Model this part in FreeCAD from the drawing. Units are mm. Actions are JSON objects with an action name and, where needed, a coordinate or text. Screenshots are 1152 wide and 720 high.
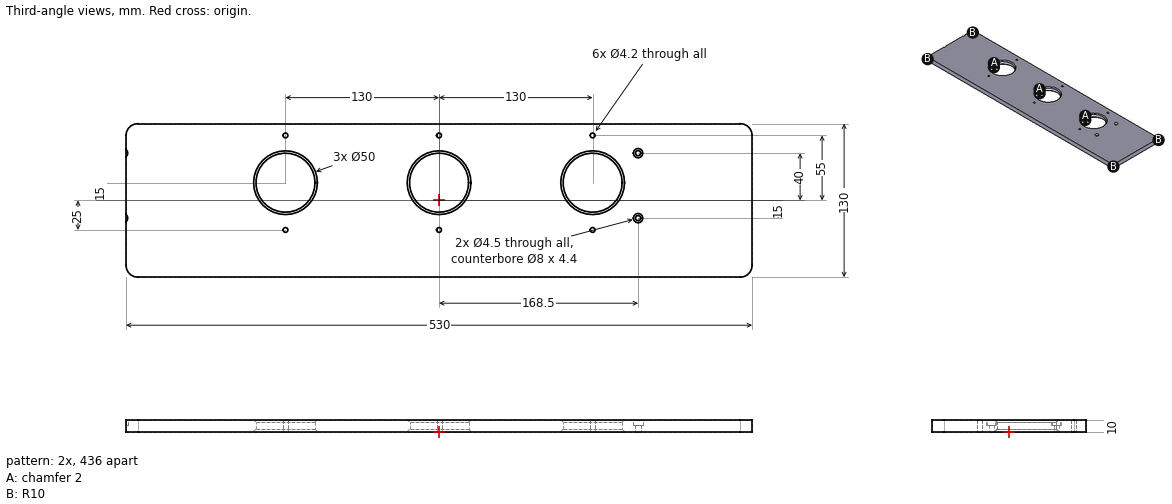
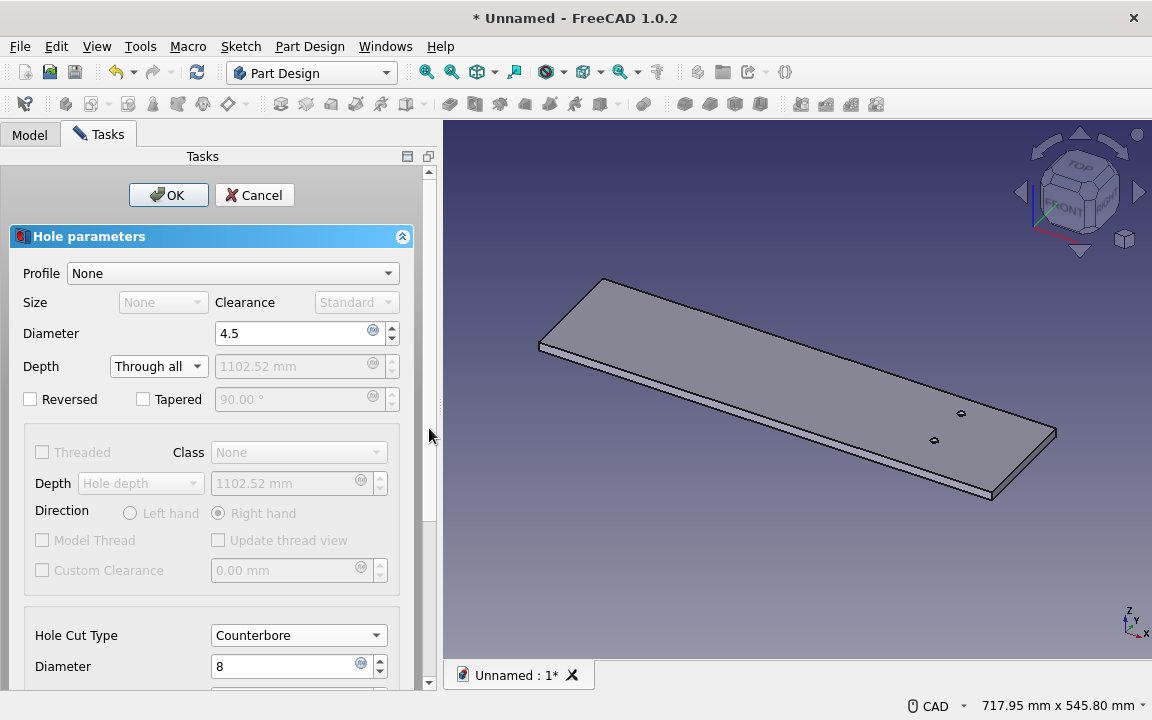
{"action": "left_click", "coordinate": [169, 195]}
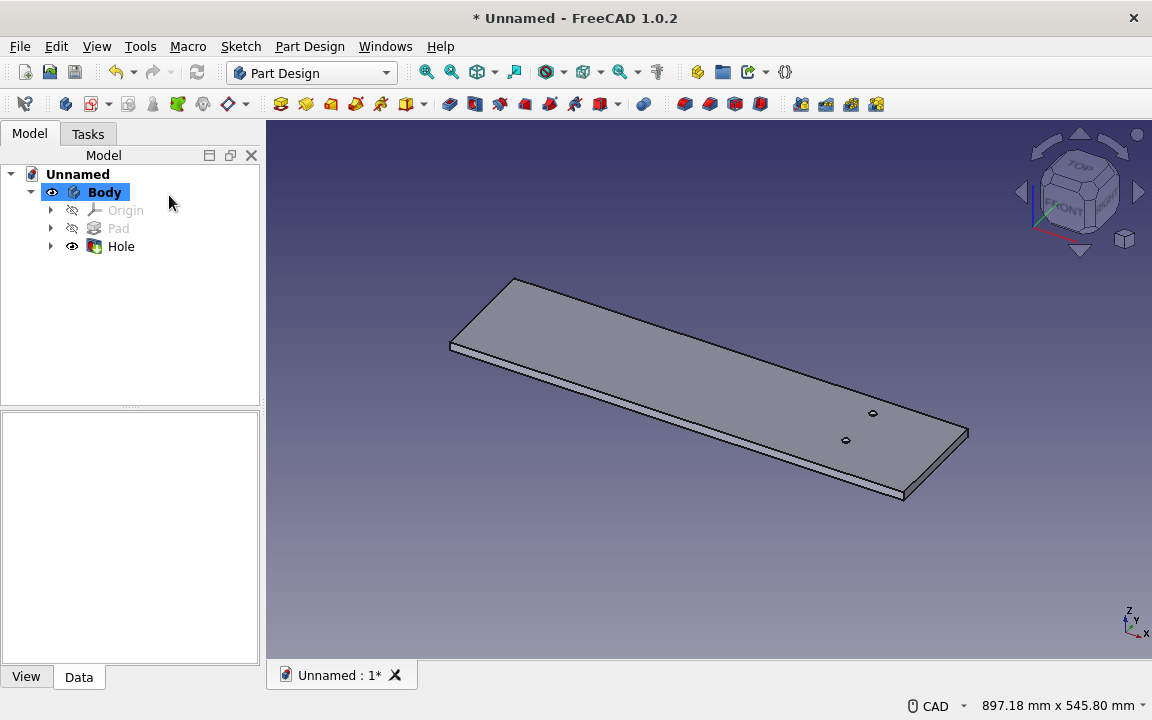
{"action": "left_click", "coordinate": [117, 246]}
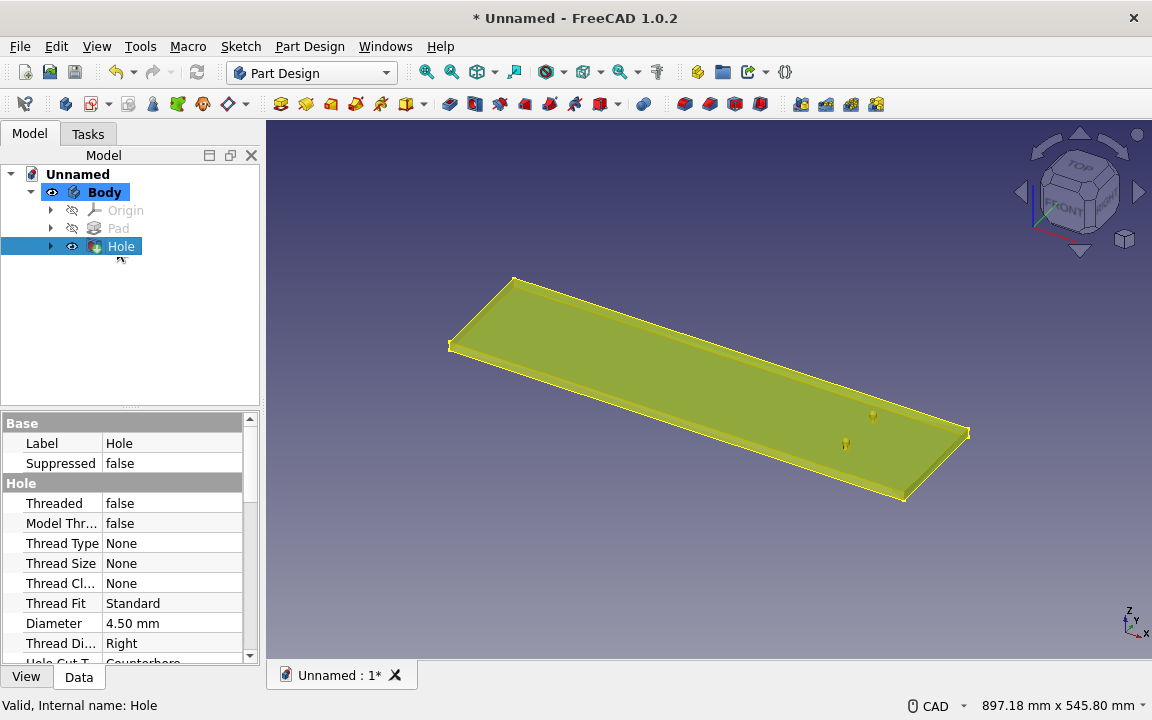
{"action": "left_click", "coordinate": [826, 104]}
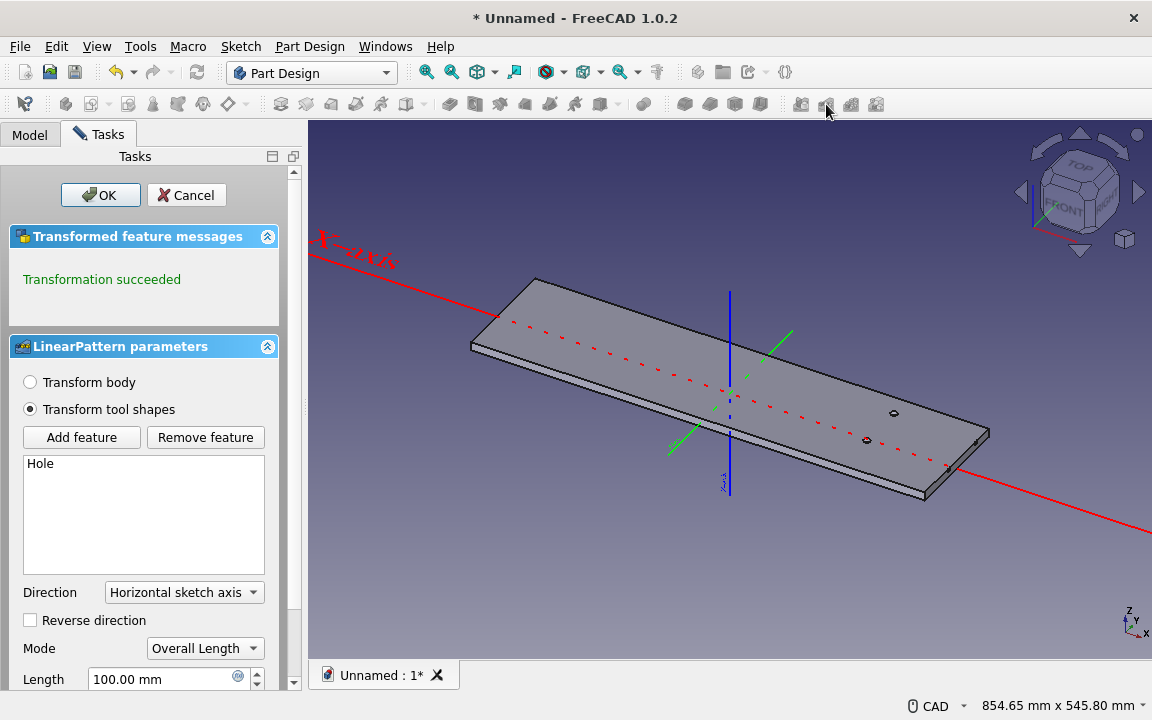
{"action": "left_click", "coordinate": [185, 592]}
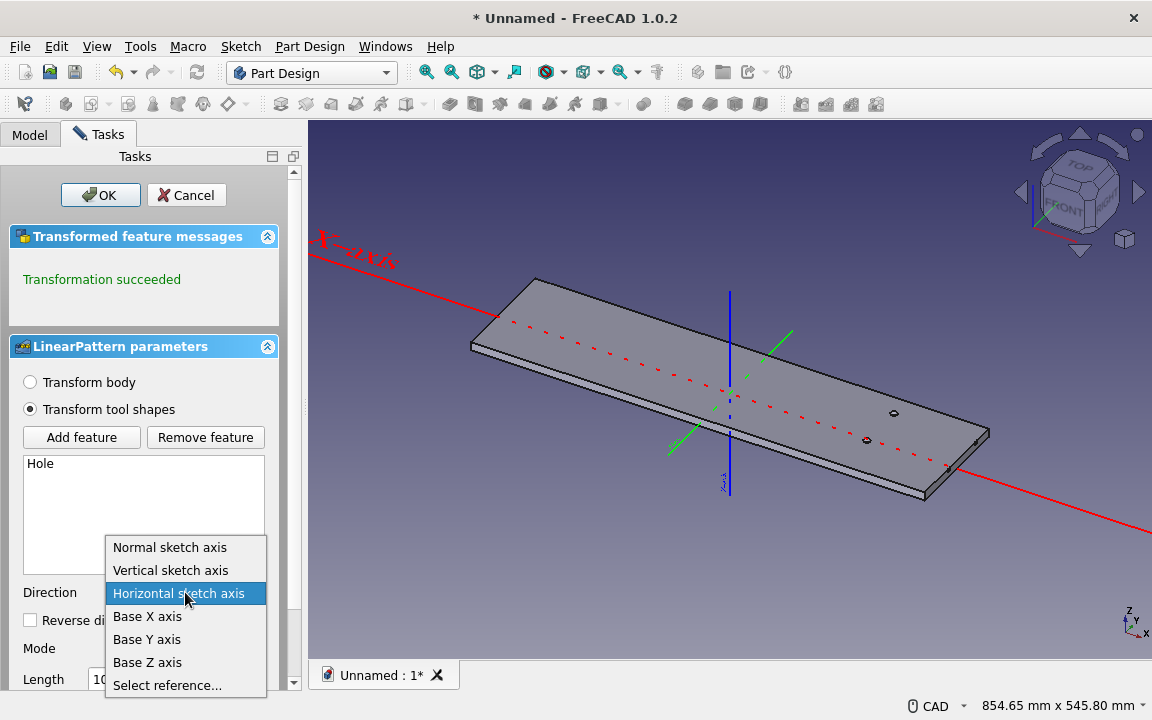
{"action": "left_click", "coordinate": [184, 616]}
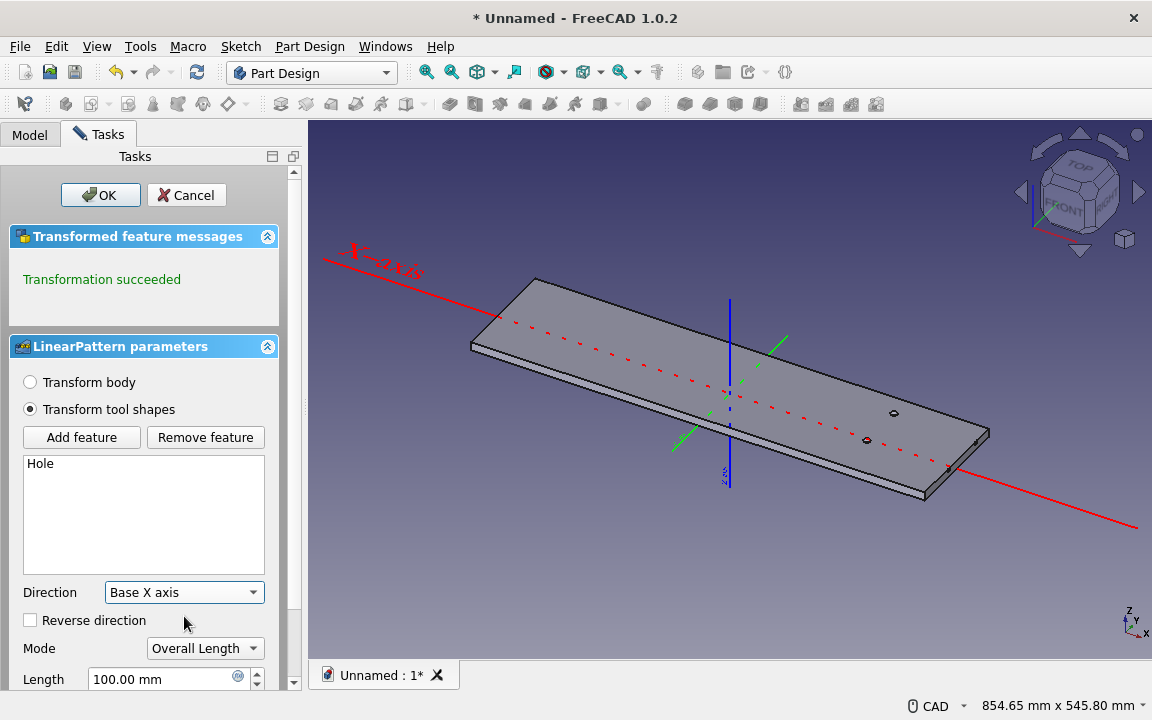
{"action": "left_click", "coordinate": [206, 648]}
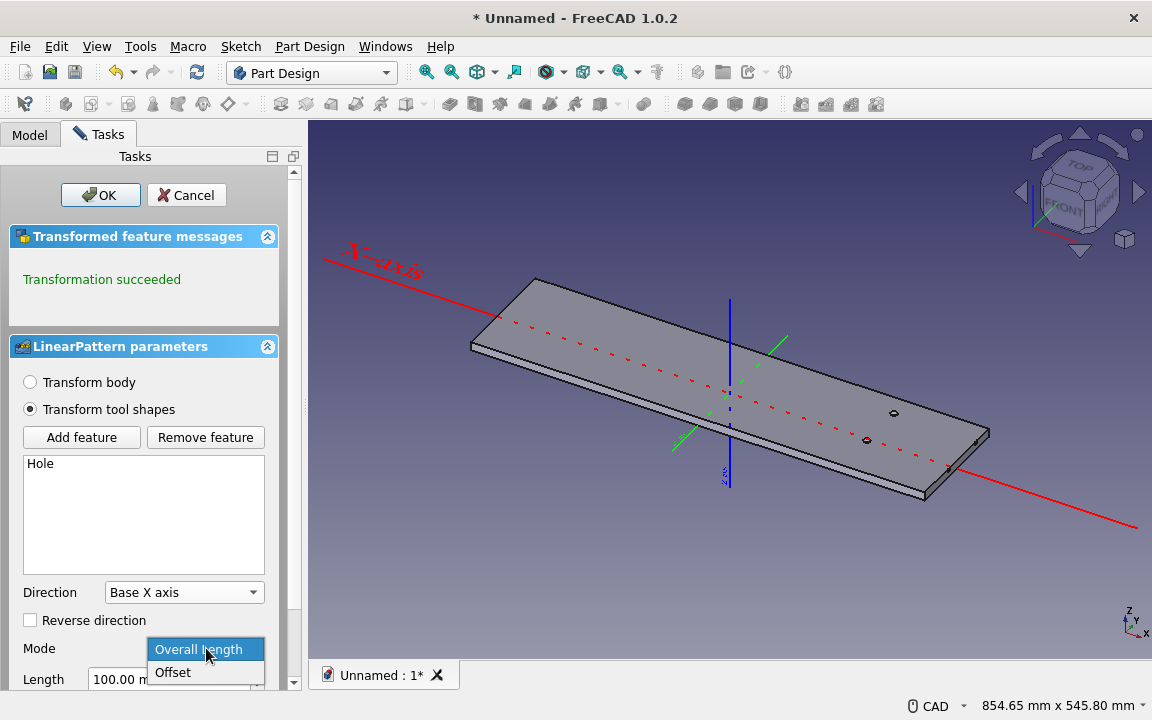
{"action": "left_click", "coordinate": [204, 672]}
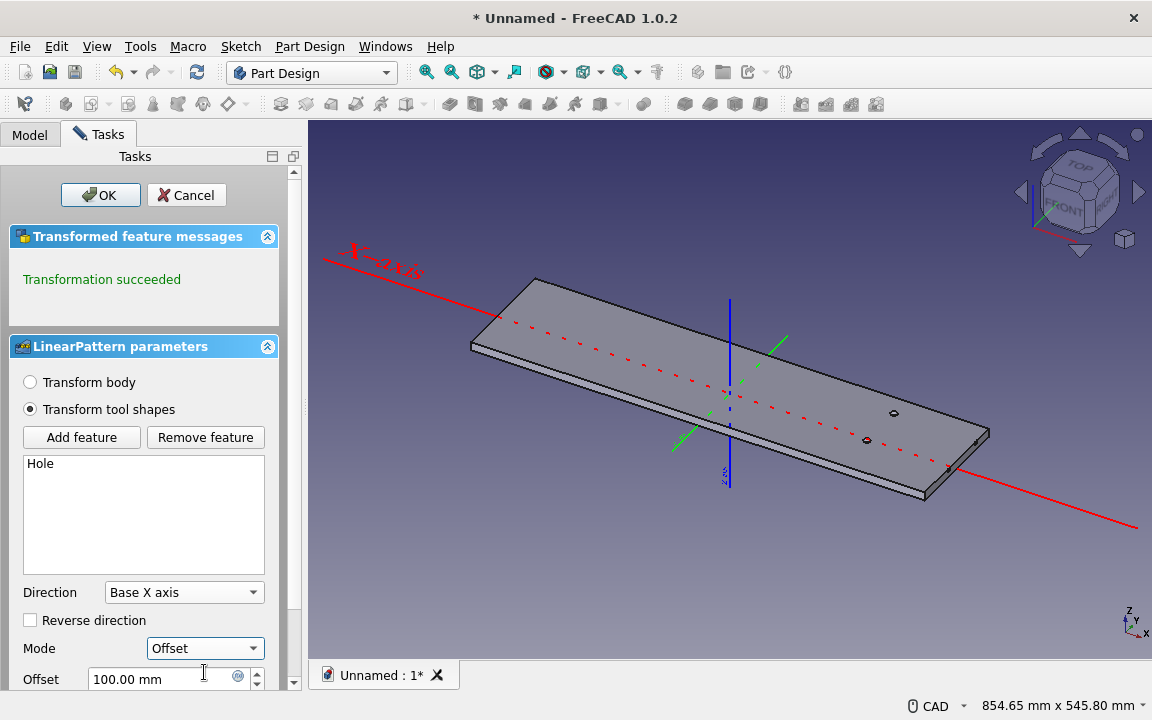
{"action": "scroll", "coordinate": [294, 428], "scroll_direction": "down", "scroll_amount": 2}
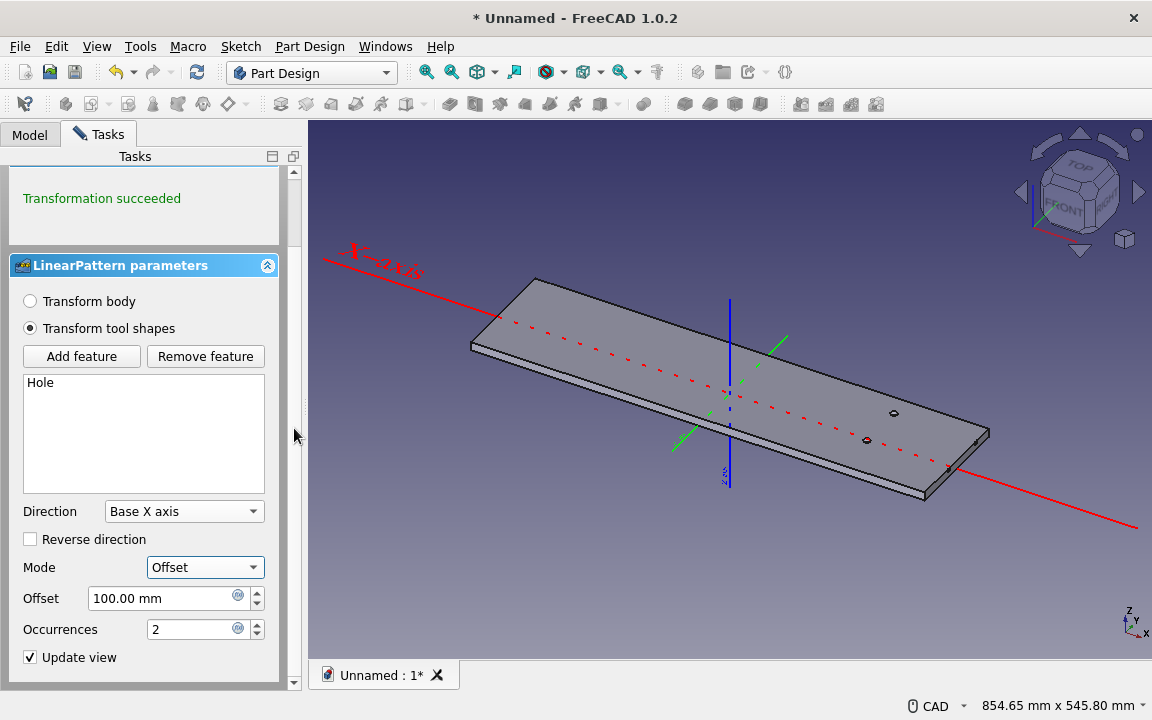
{"action": "triple_click", "coordinate": [170, 598]}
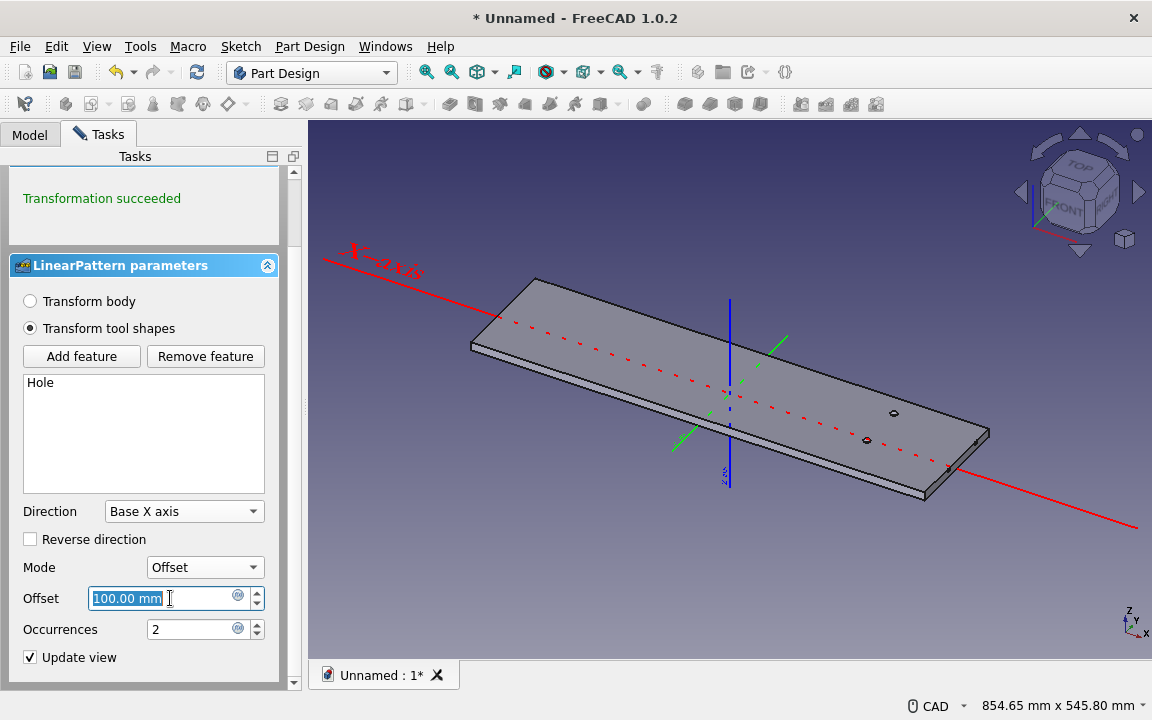
{"action": "type", "text": "436"}
{"action": "key", "text": "Tab"}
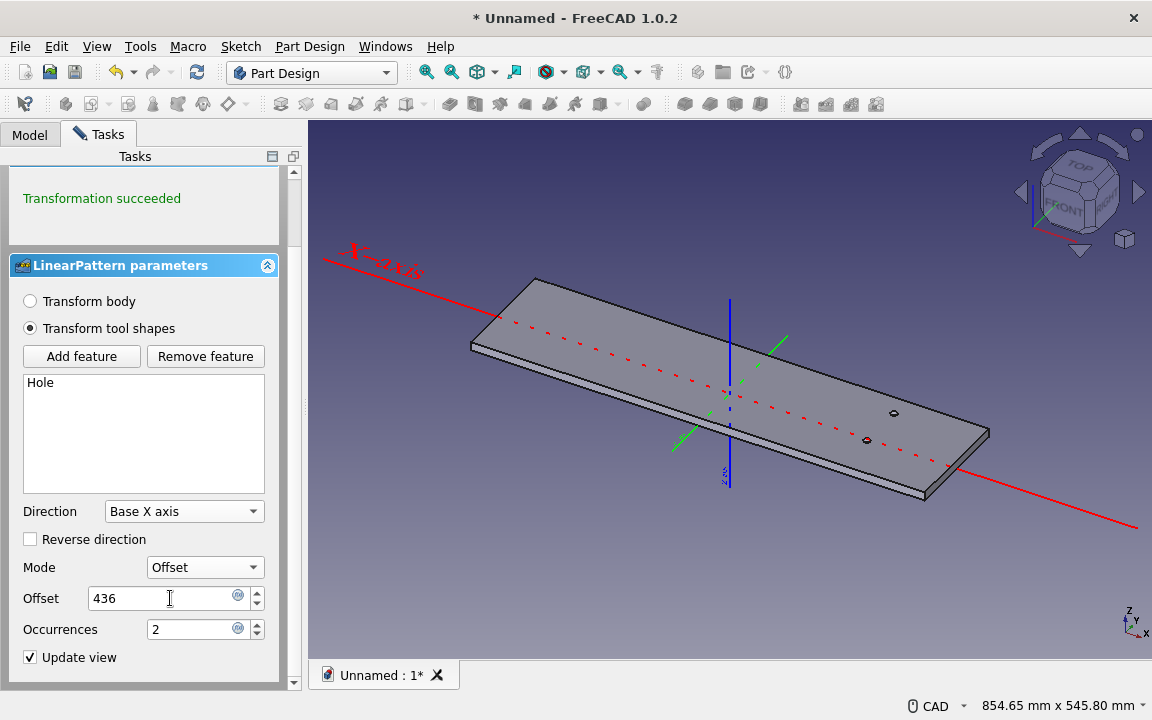
{"action": "triple_click", "coordinate": [199, 630]}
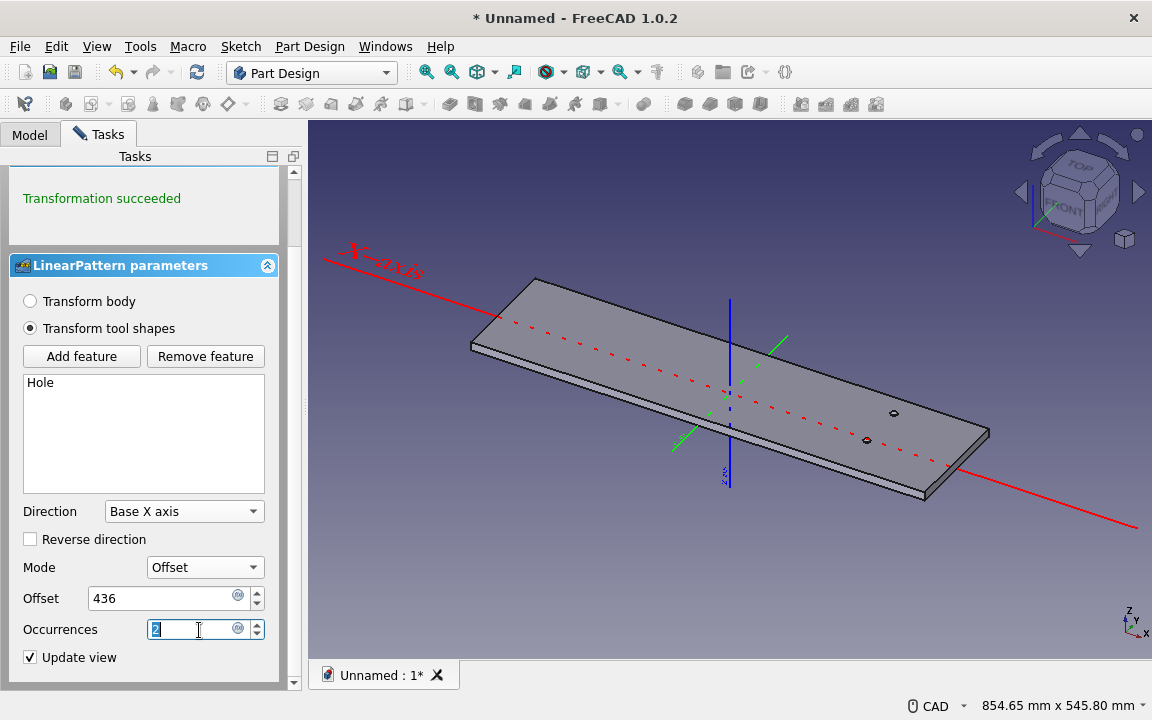
{"action": "type", "text": "2"}
{"action": "key", "text": "Tab"}